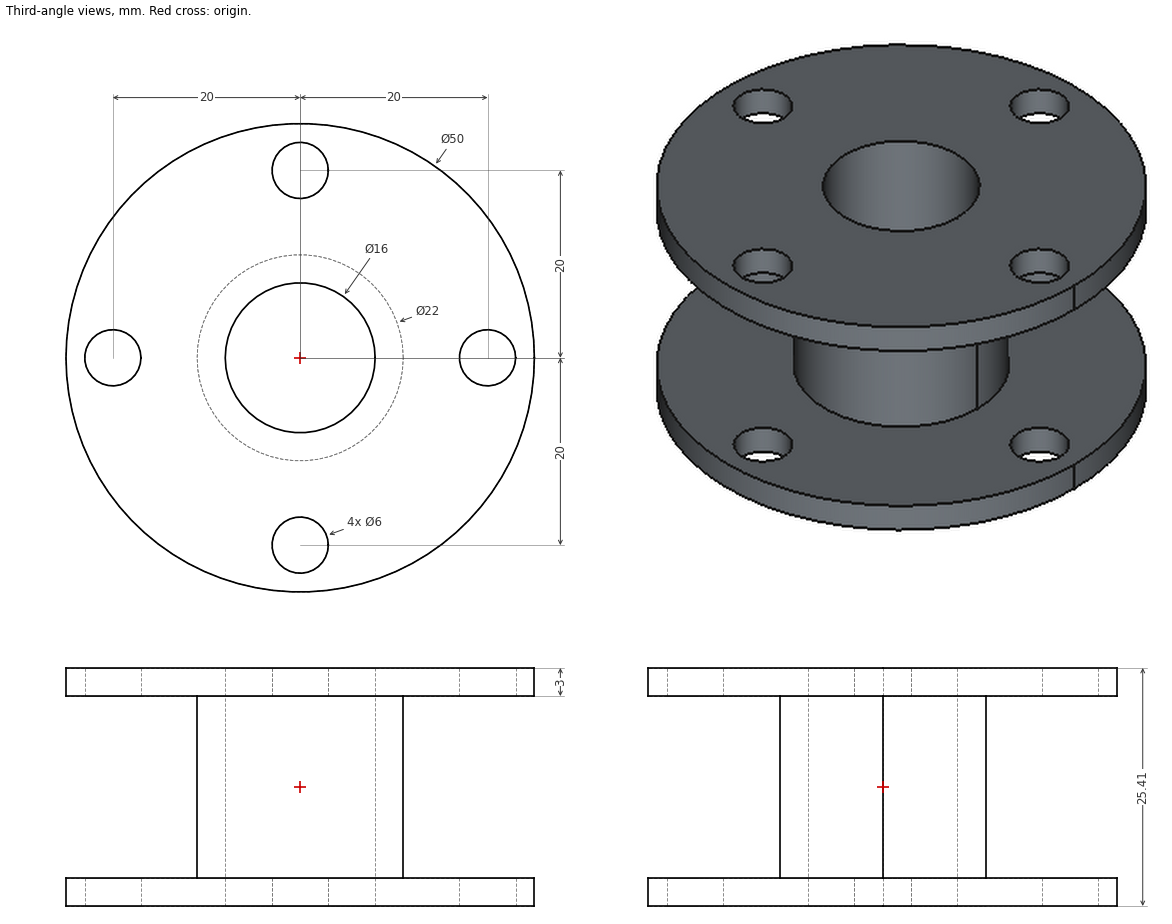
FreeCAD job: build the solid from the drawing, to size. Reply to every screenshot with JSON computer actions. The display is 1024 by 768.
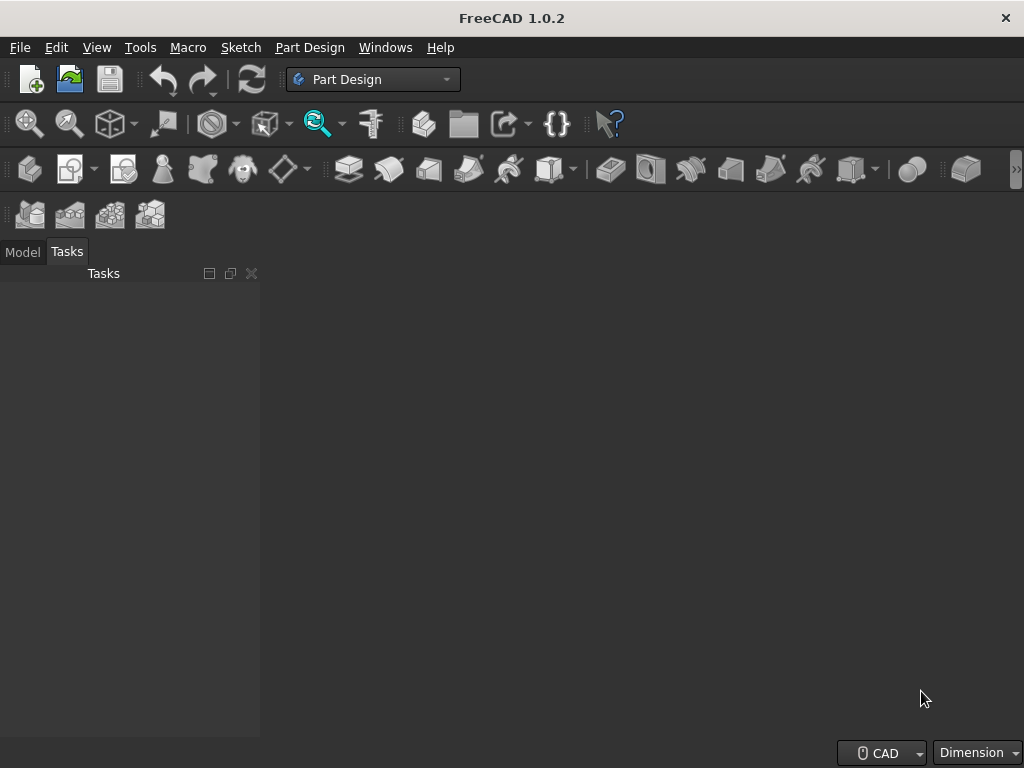
{"action": "key", "text": "ctrl+n"}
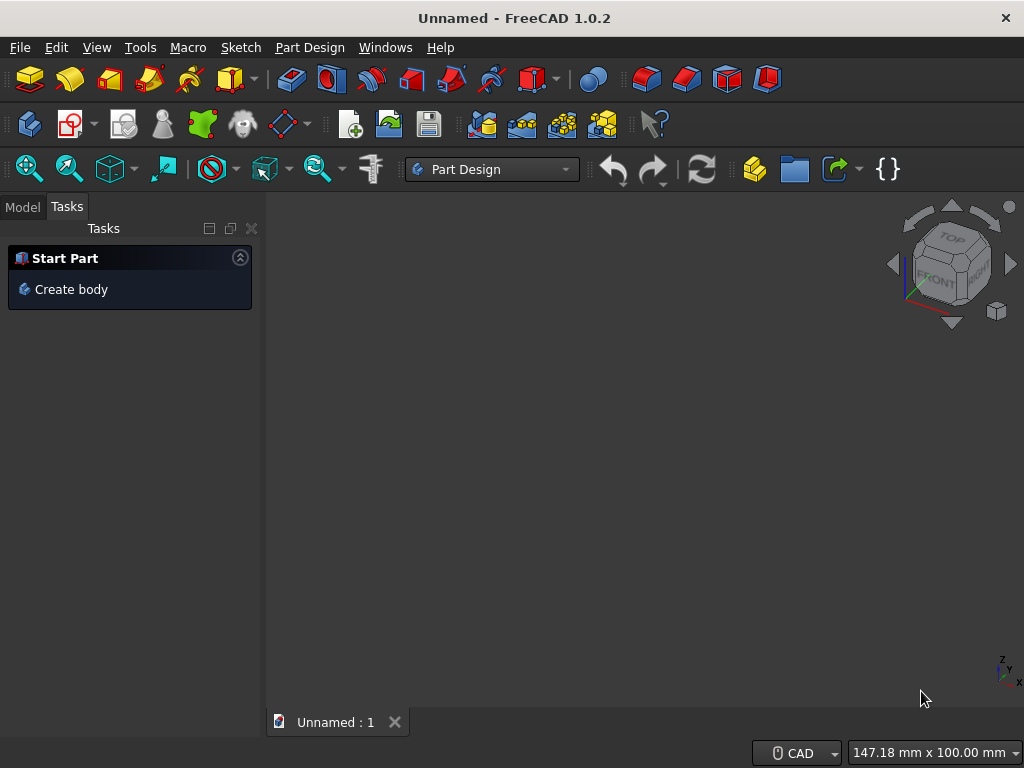
{"action": "left_click", "coordinate": [70, 124]}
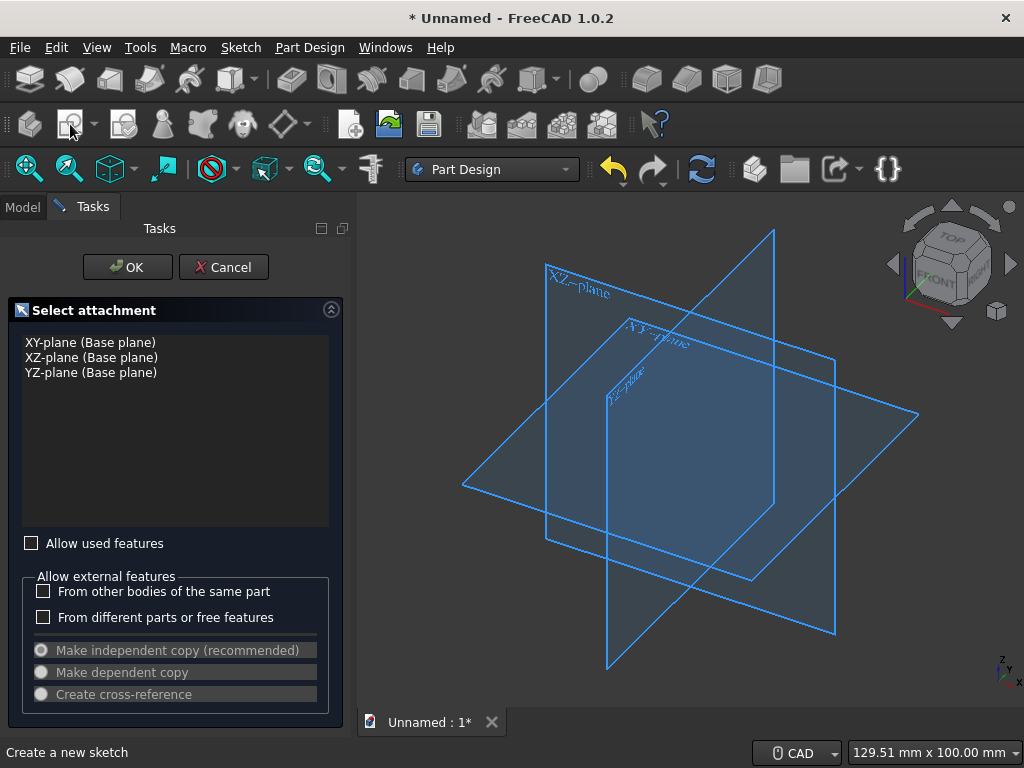
{"action": "left_click", "coordinate": [82, 342]}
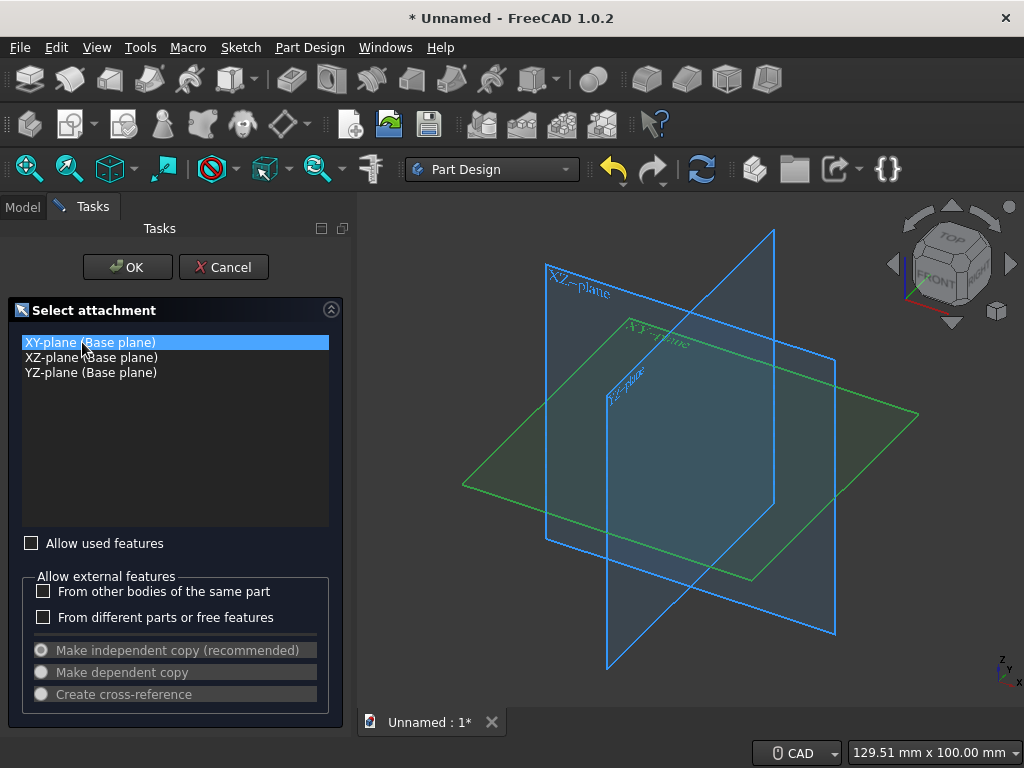
{"action": "left_click", "coordinate": [128, 267]}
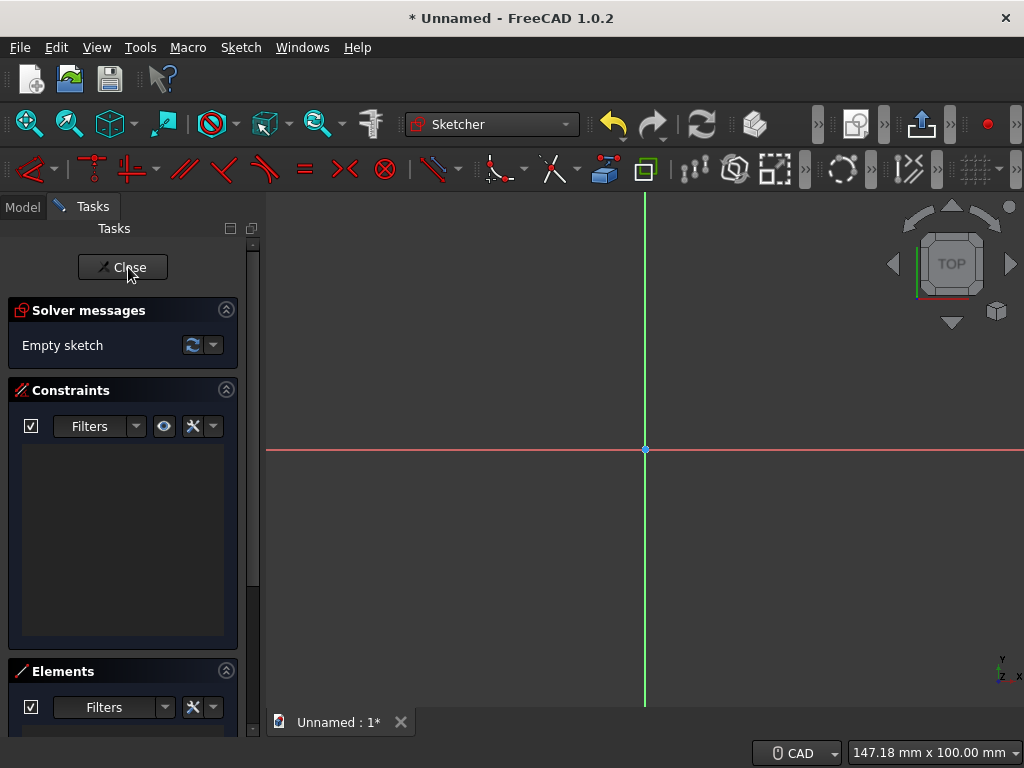
{"action": "scroll", "coordinate": [685, 449], "scroll_direction": "up", "scroll_amount": 5}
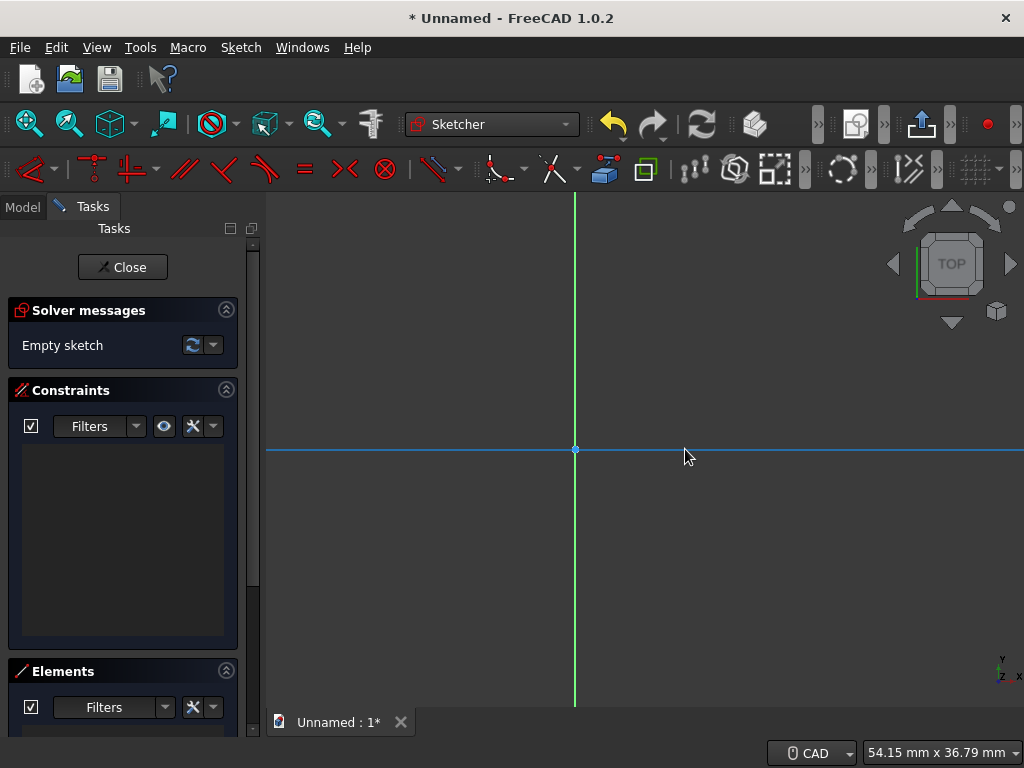
{"action": "key", "text": "g c"}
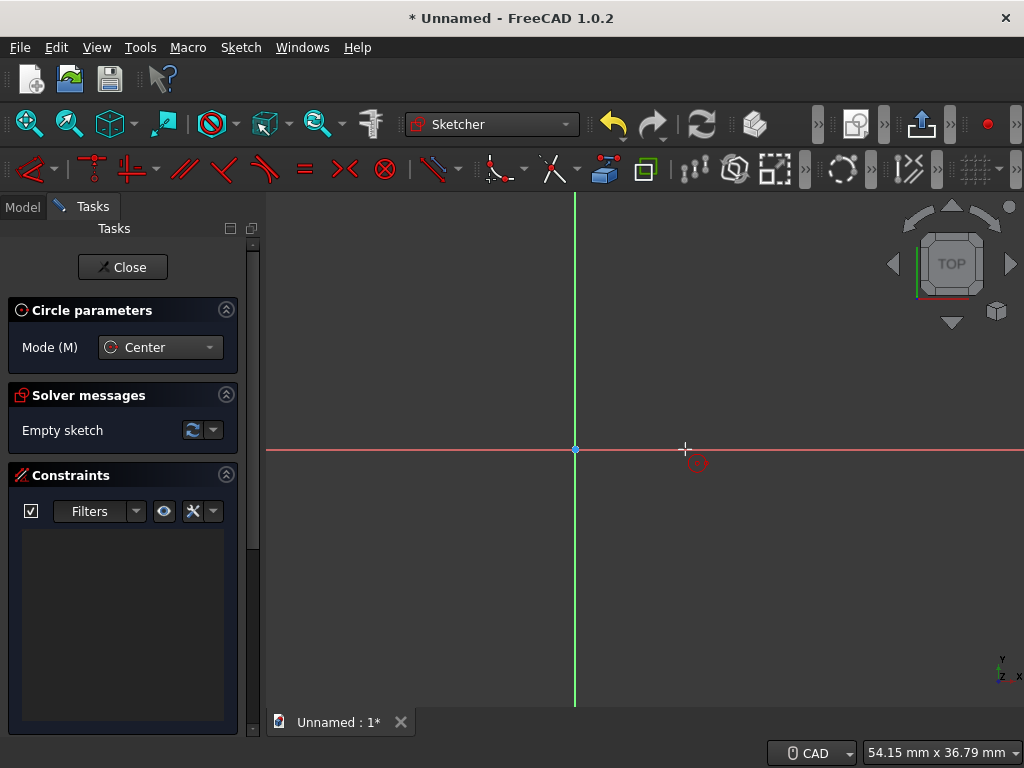
{"action": "left_click", "coordinate": [575, 450]}
{"action": "left_click", "coordinate": [684, 341]}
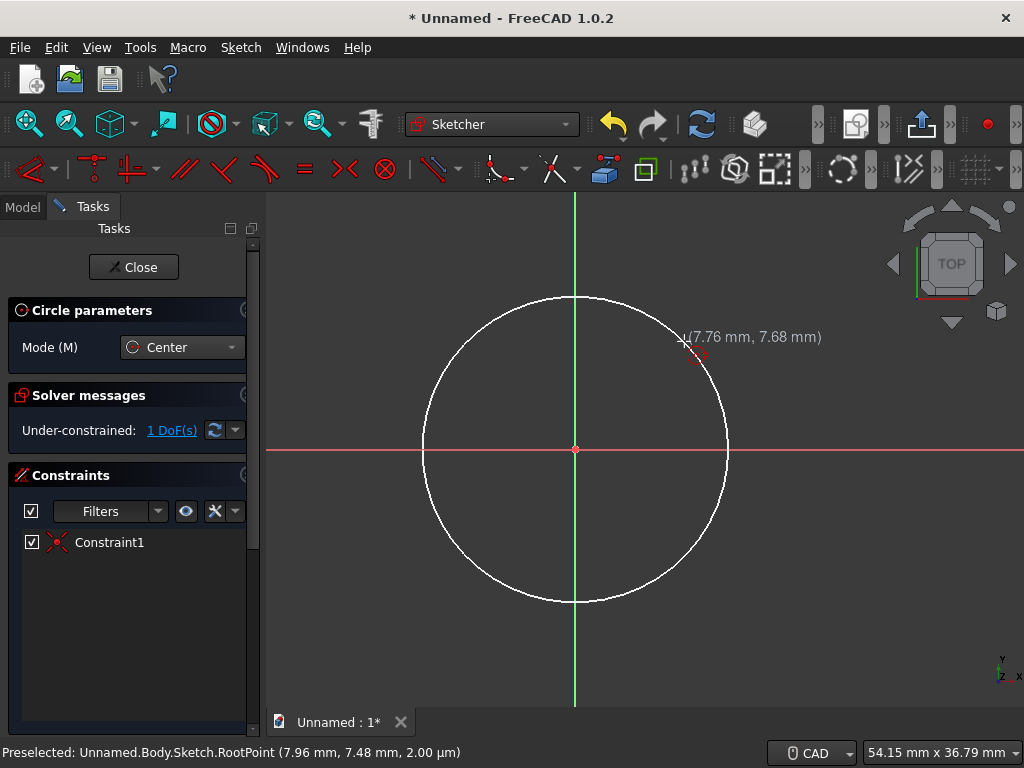
{"action": "left_click", "coordinate": [575, 450]}
{"action": "left_click", "coordinate": [655, 370]}
{"action": "key", "text": "Escape"}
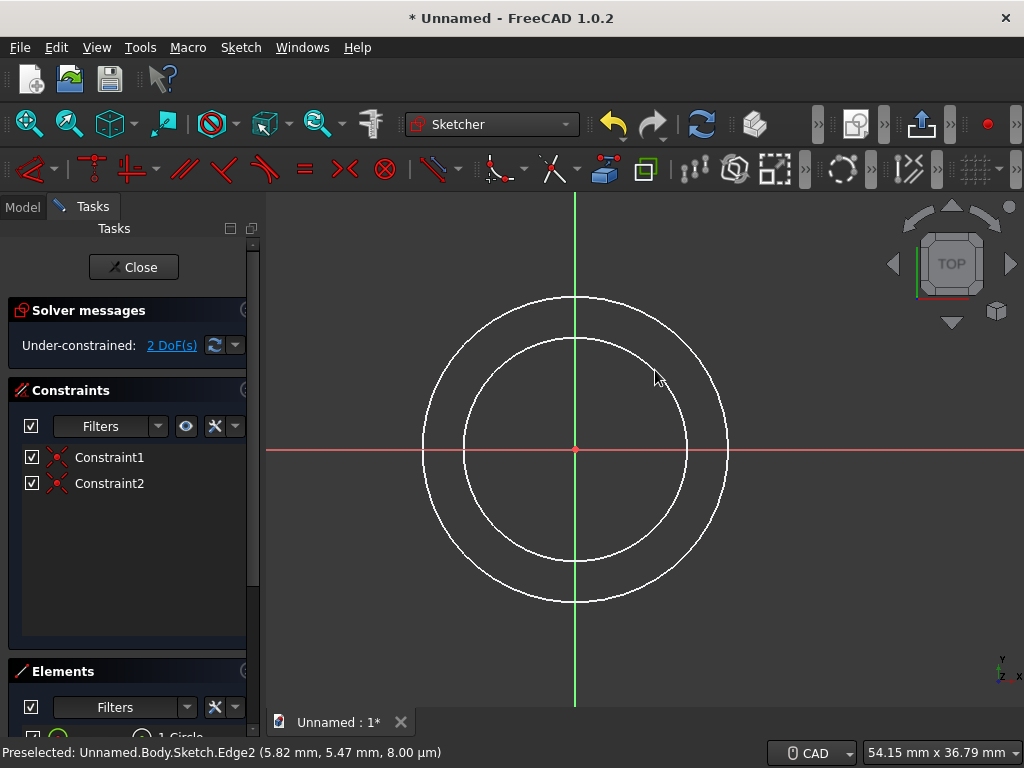
{"action": "left_click", "coordinate": [683, 341]}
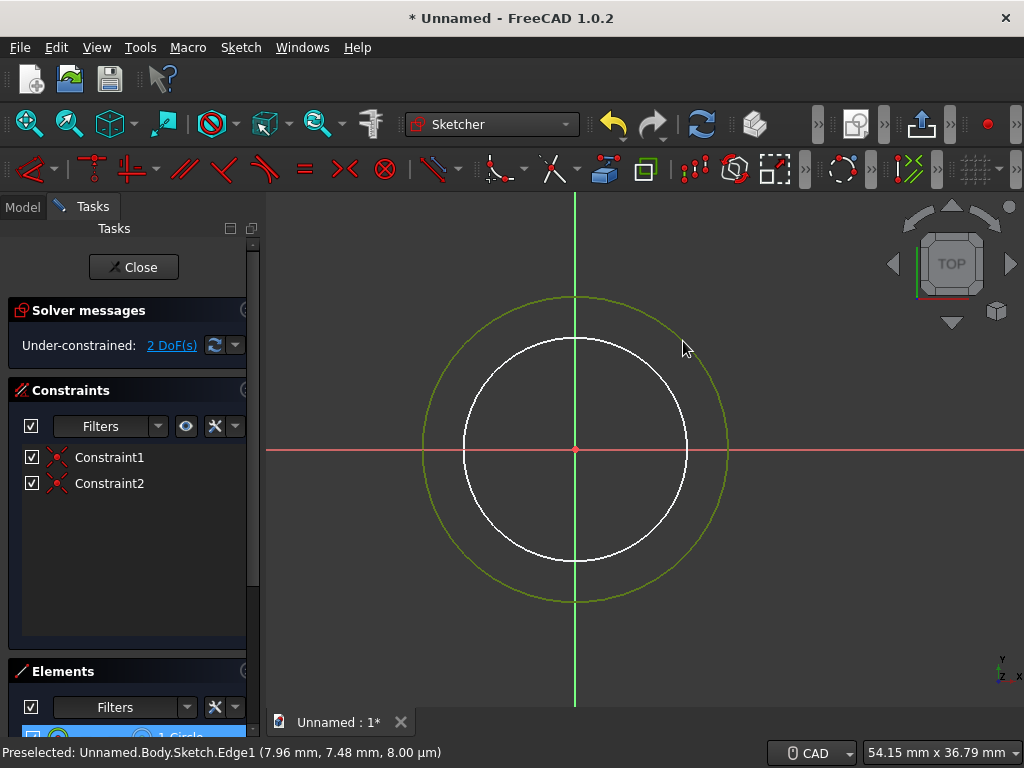
{"action": "left_click", "coordinate": [56, 170]}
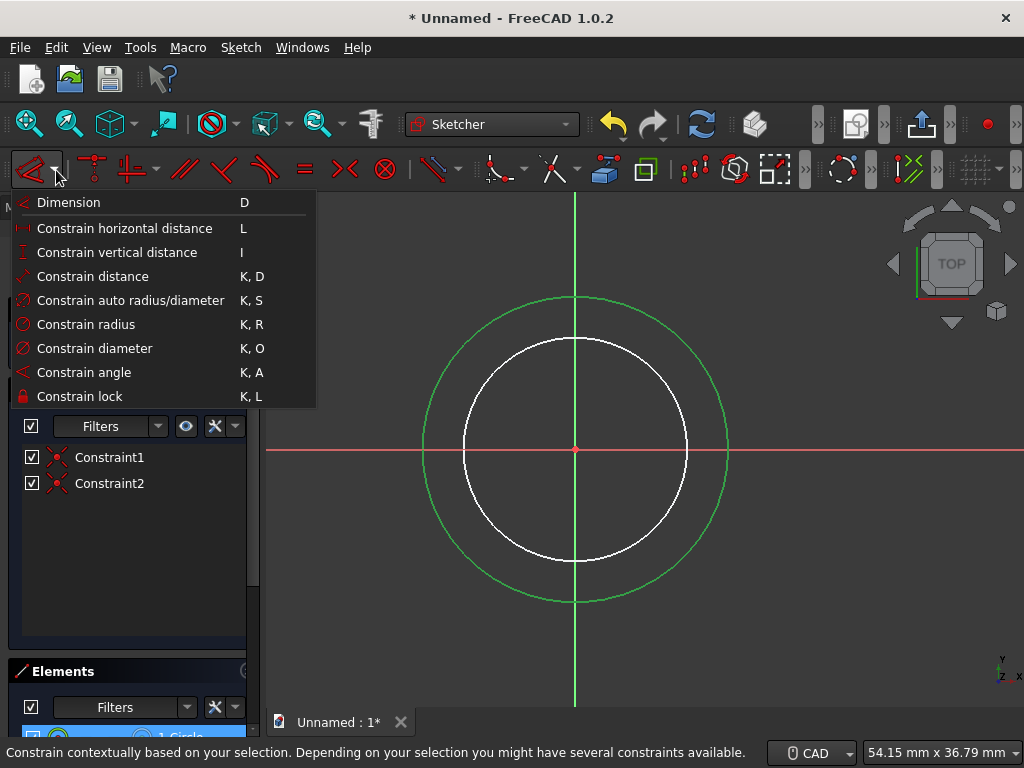
{"action": "left_click", "coordinate": [164, 348]}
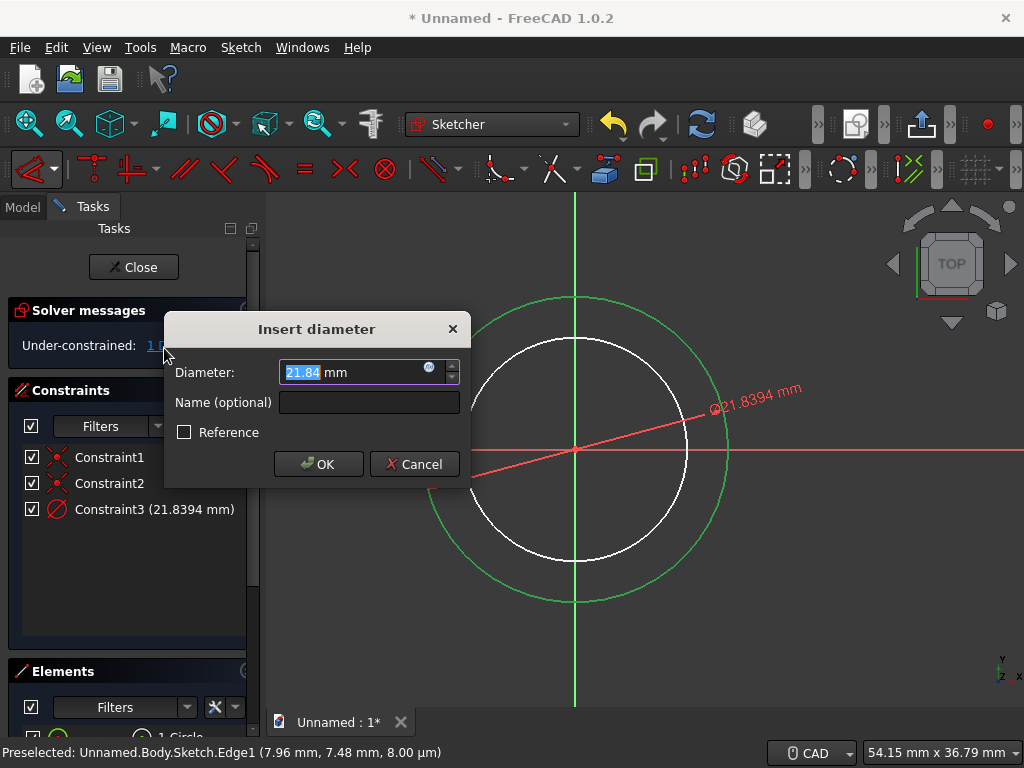
{"action": "type", "text": "22"}
{"action": "key", "text": "Return"}